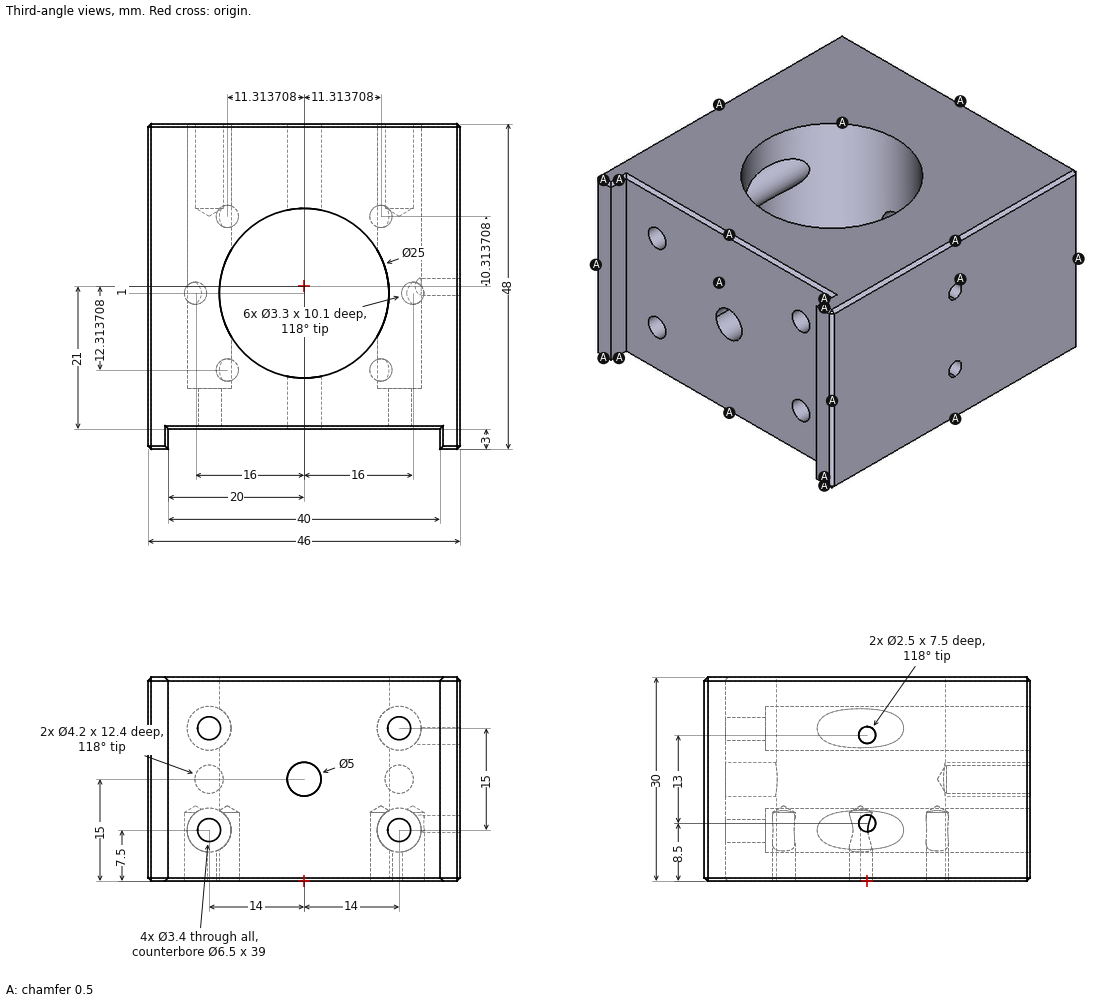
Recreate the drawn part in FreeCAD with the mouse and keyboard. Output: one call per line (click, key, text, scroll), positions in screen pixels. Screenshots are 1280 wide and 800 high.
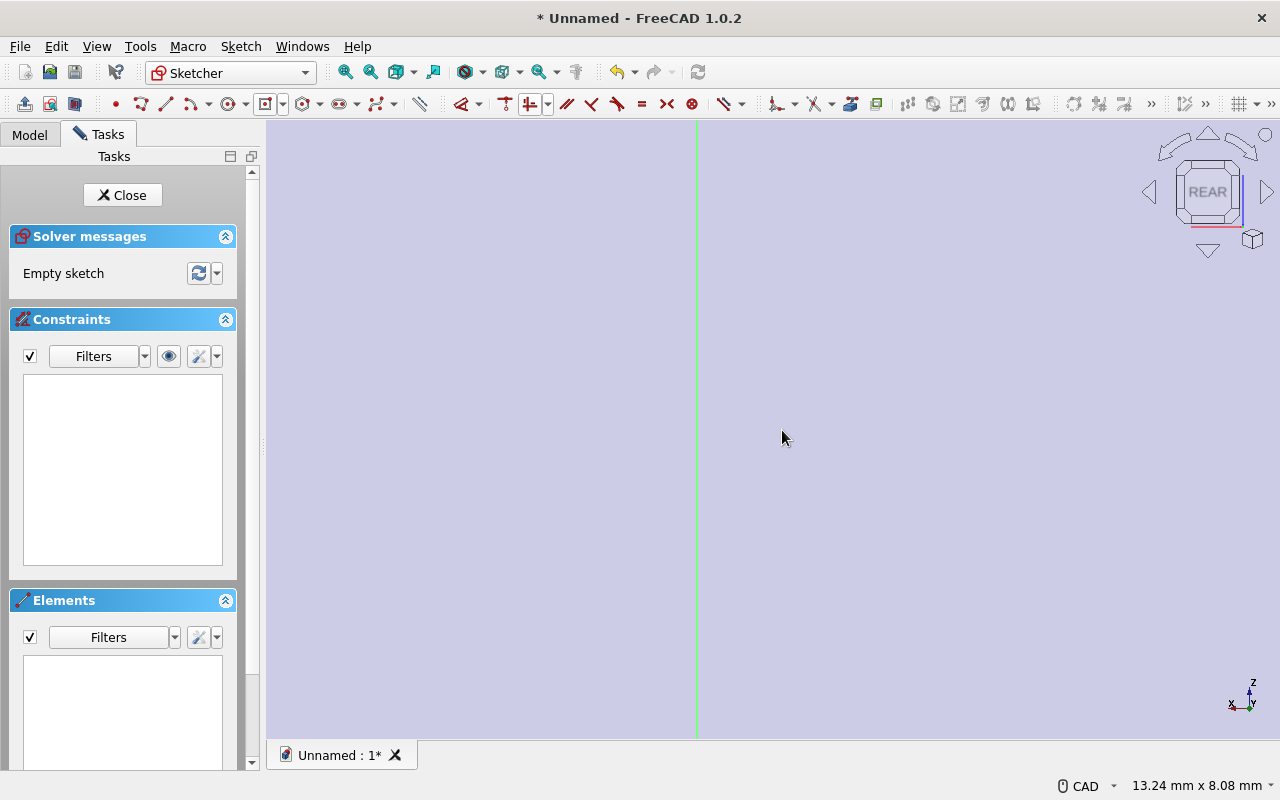
click(228, 104)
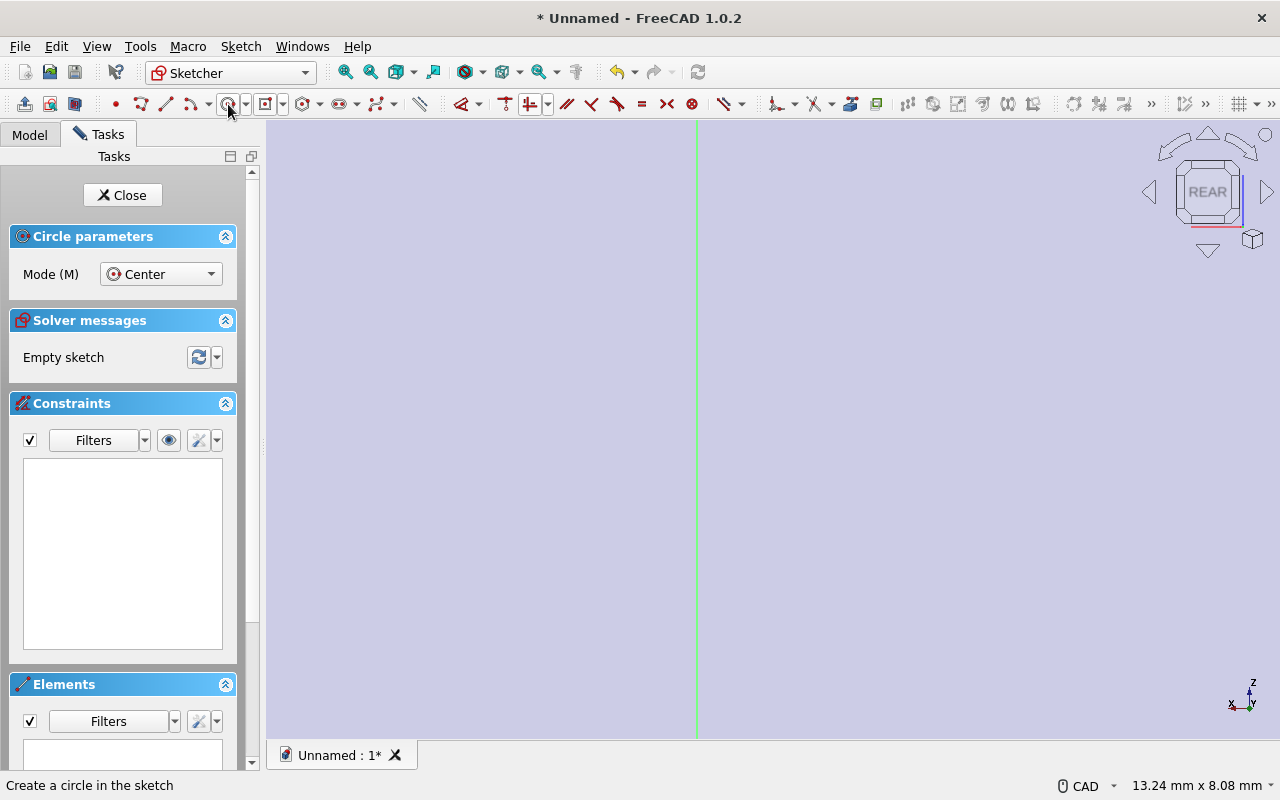
click(697, 421)
move(832, 286)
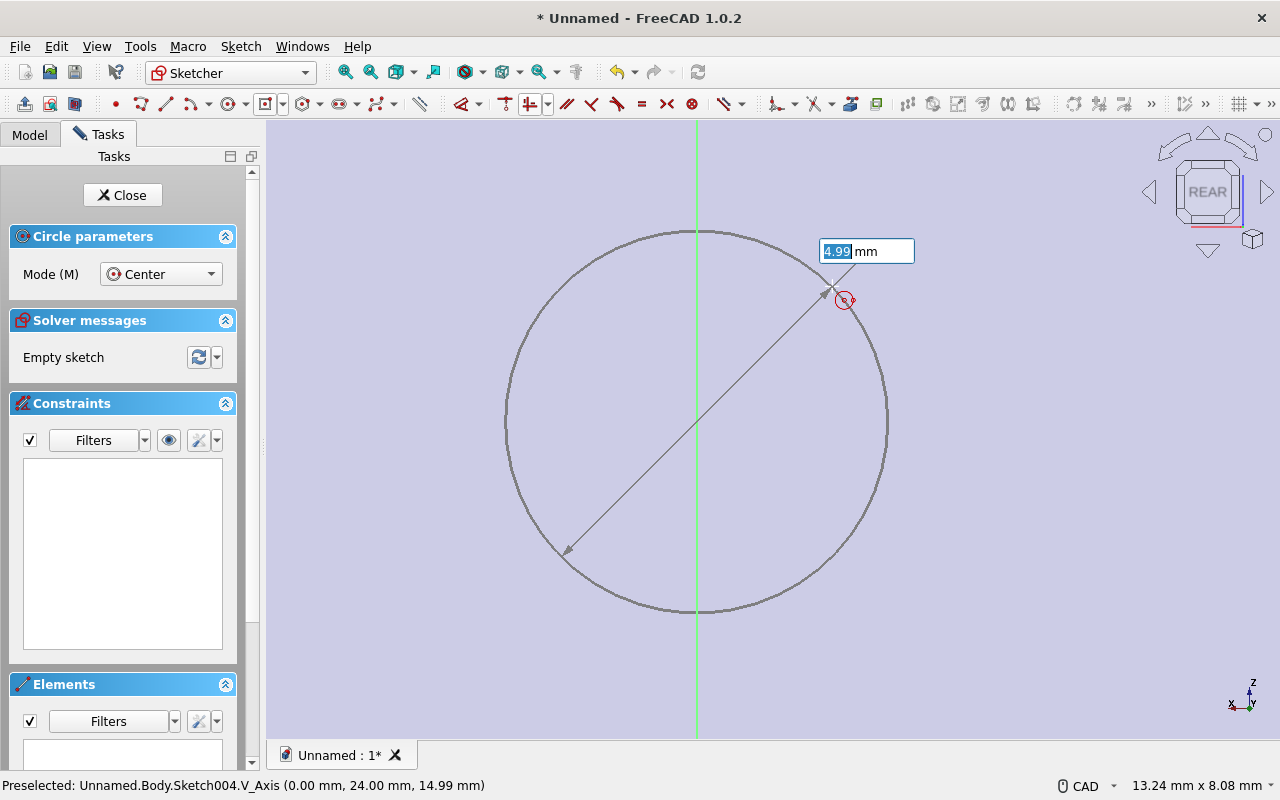
text(5)
key(Return)
key(Escape)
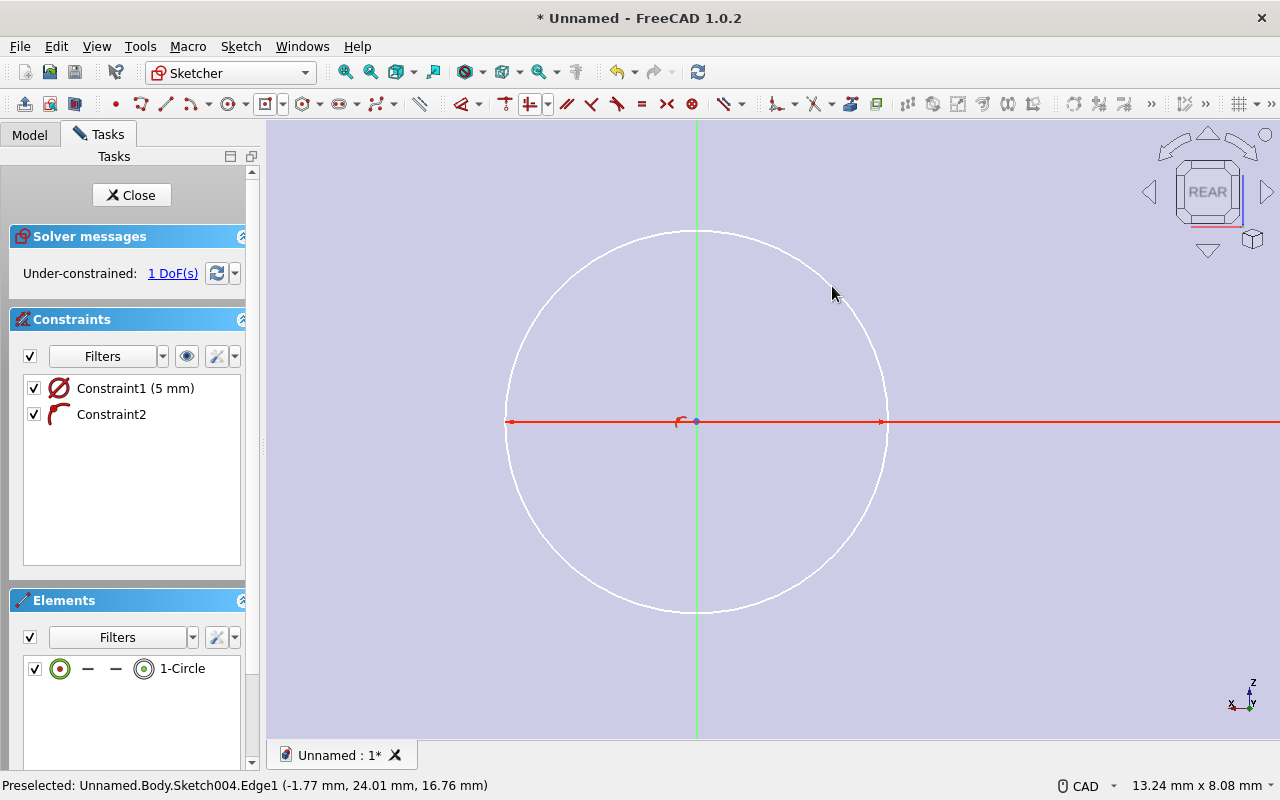
click(460, 104)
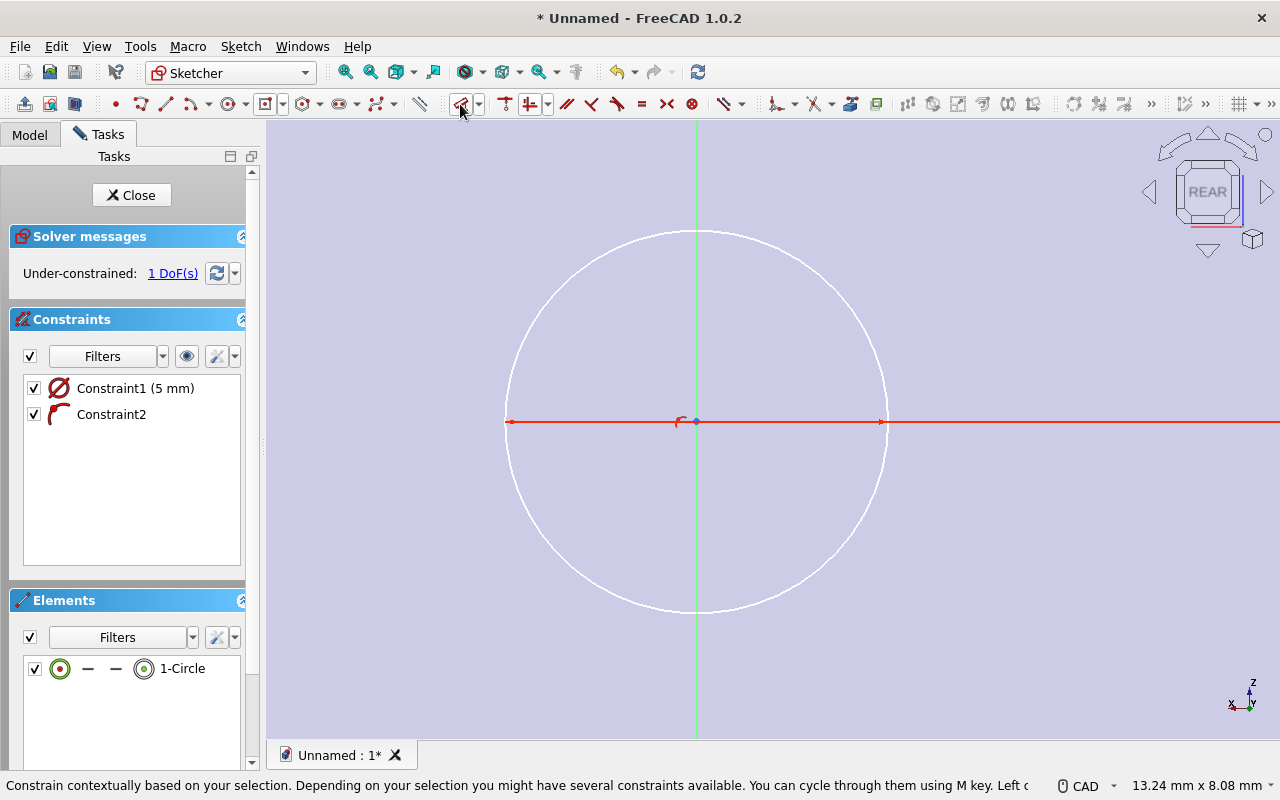
click(697, 422)
click(731, 567)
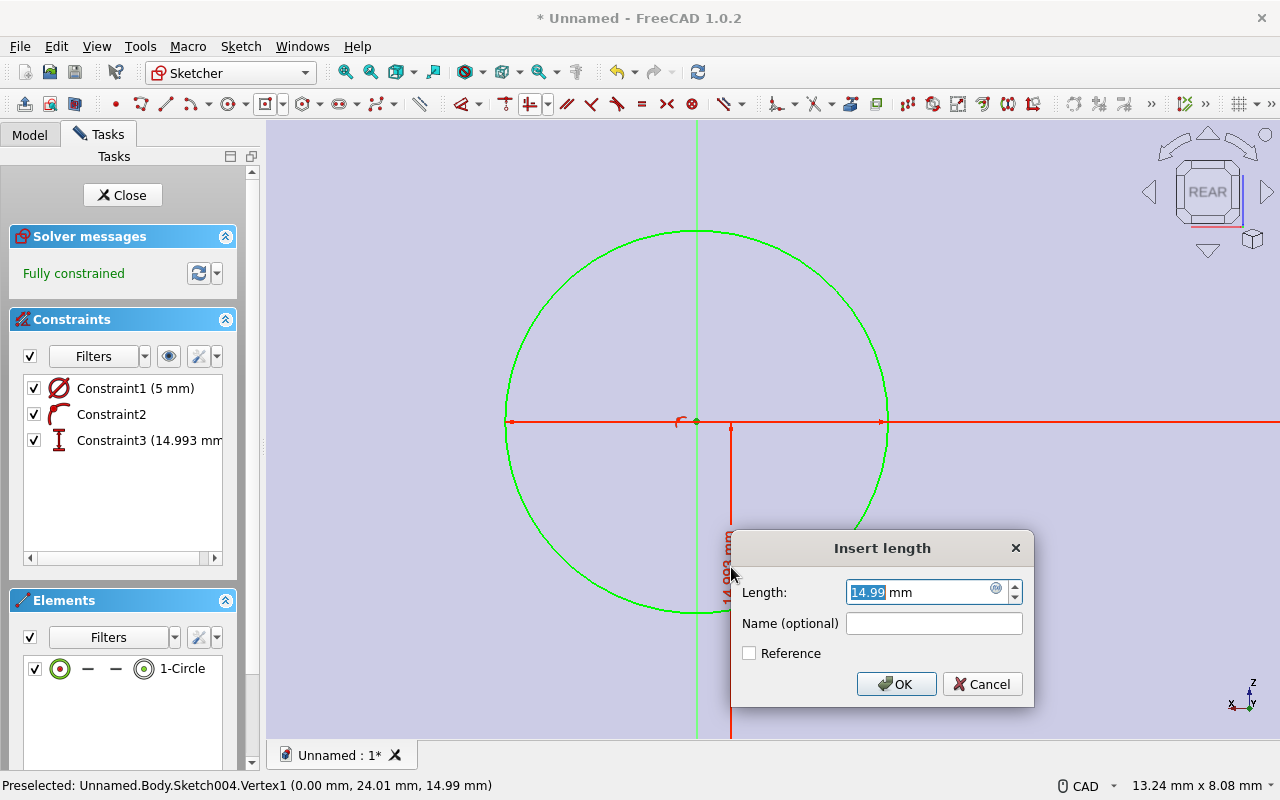
text(15)
key(Return)
key(Escape)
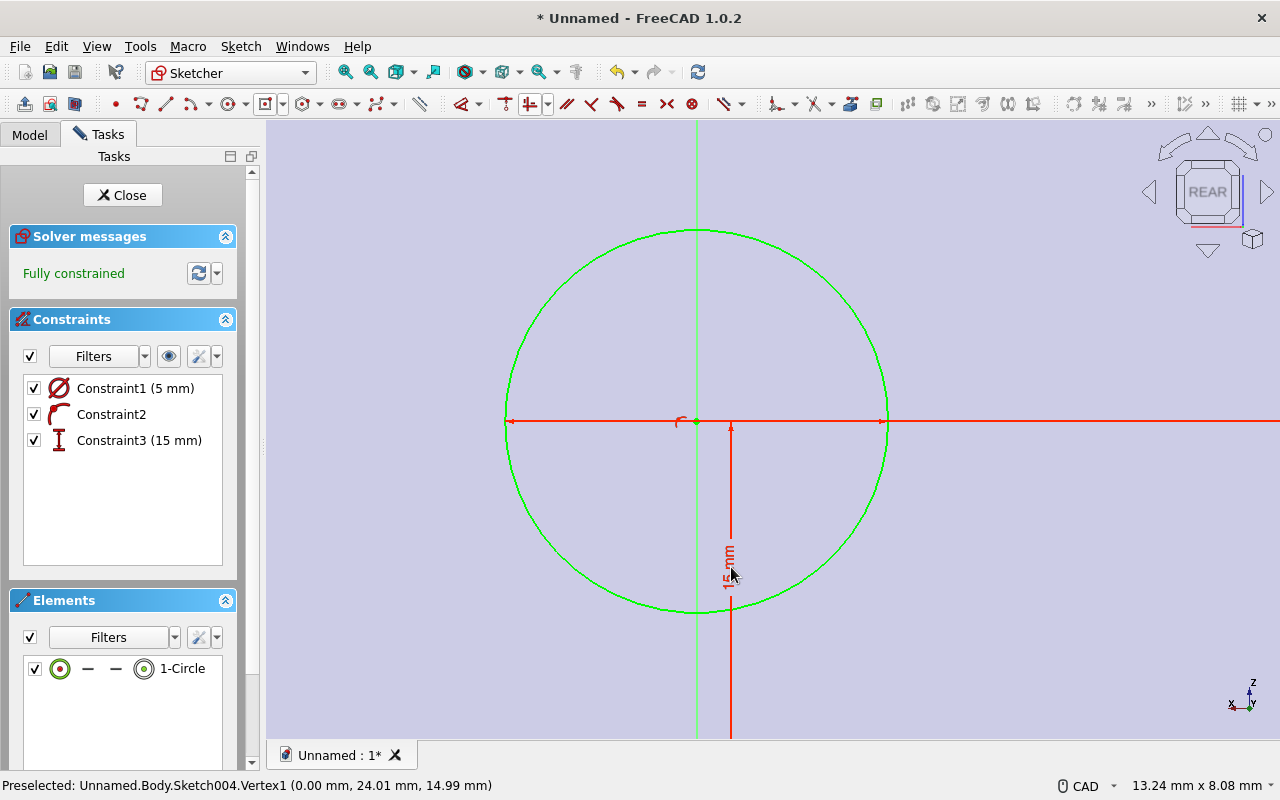
click(123, 195)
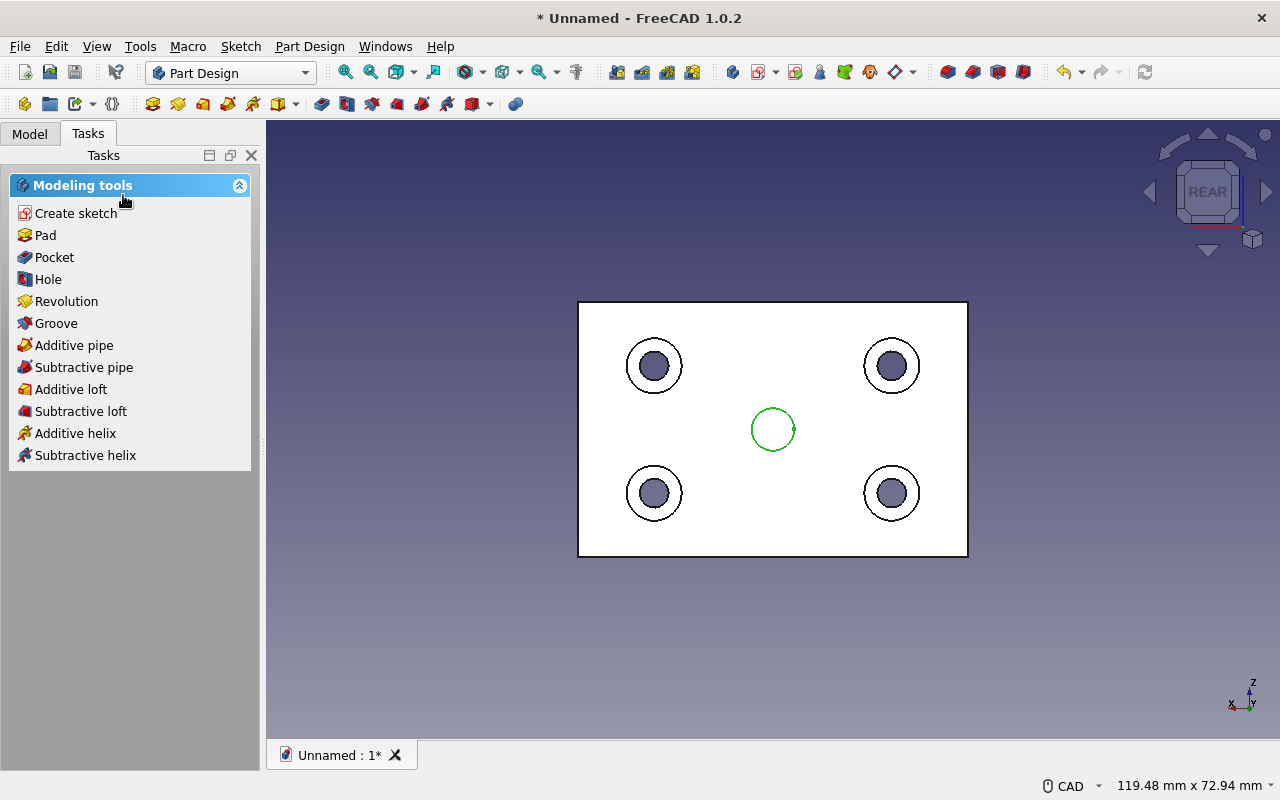
click(322, 104)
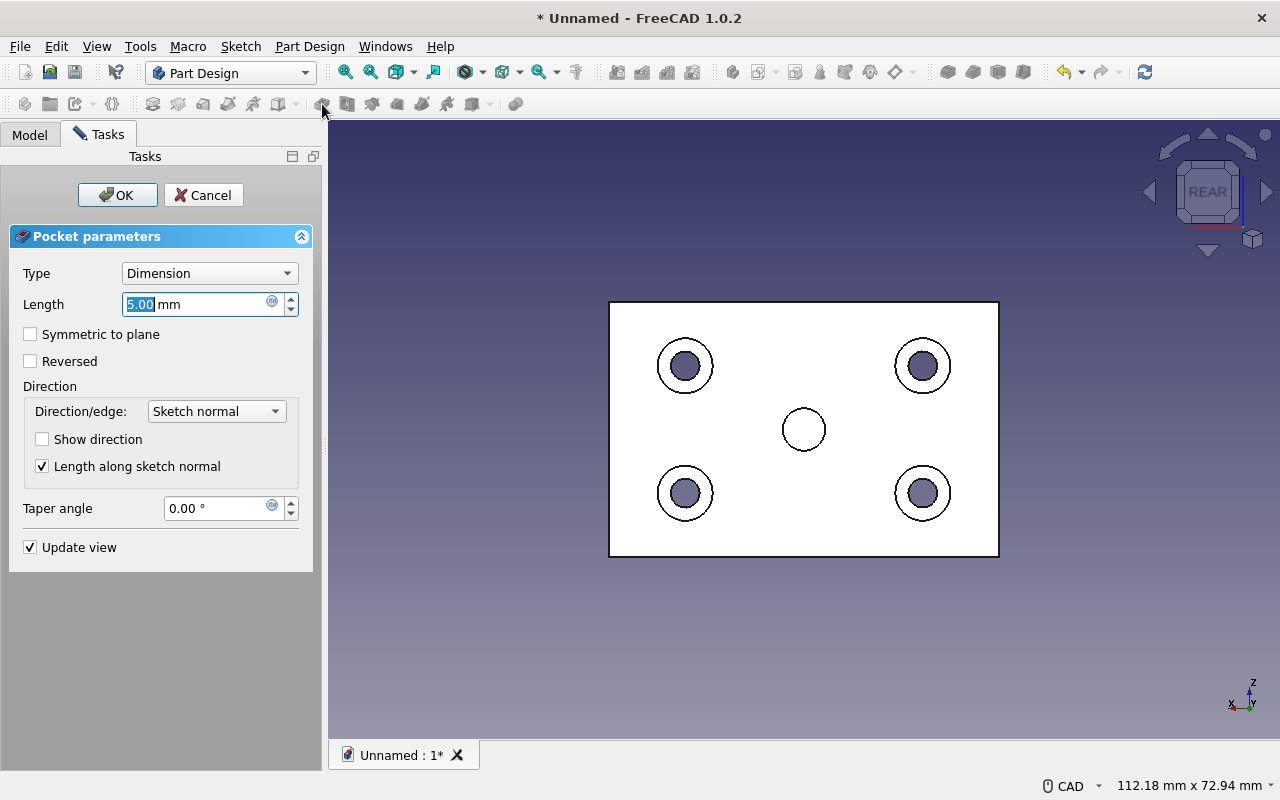
click(210, 274)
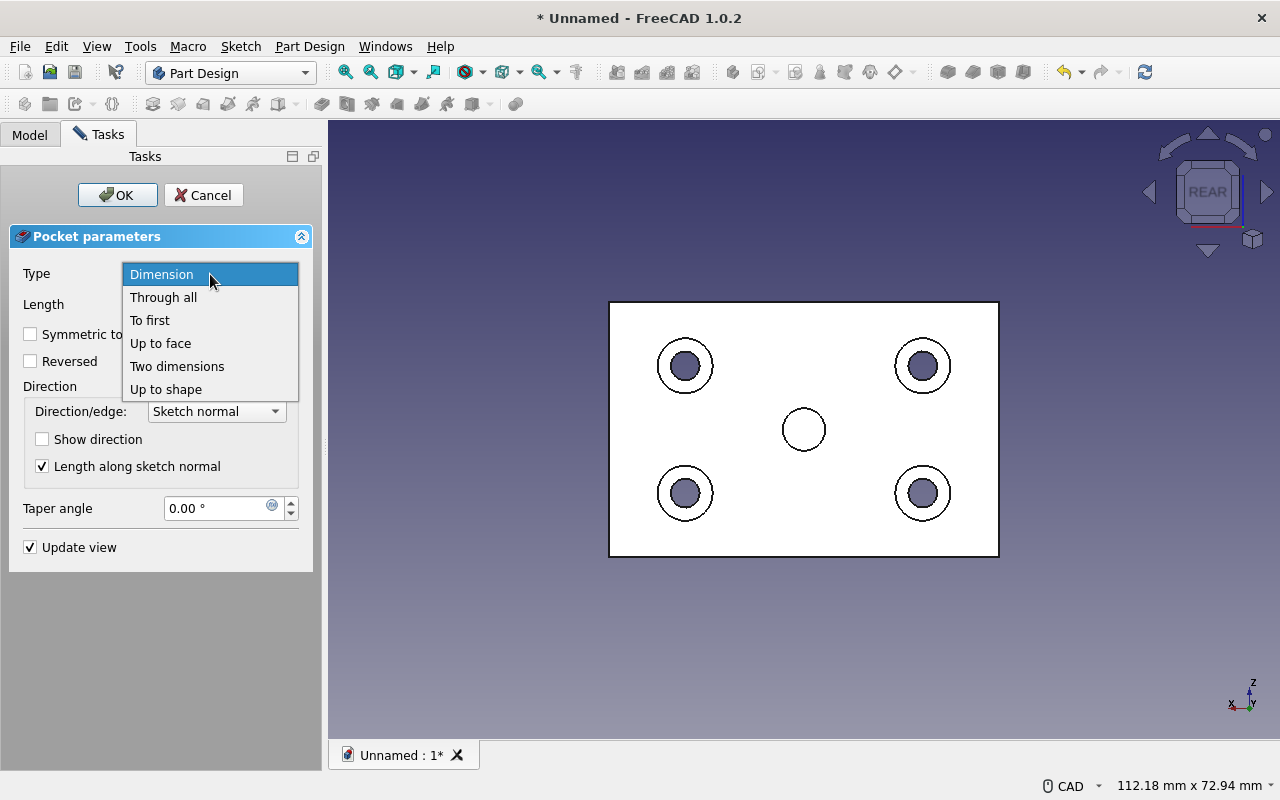
click(208, 298)